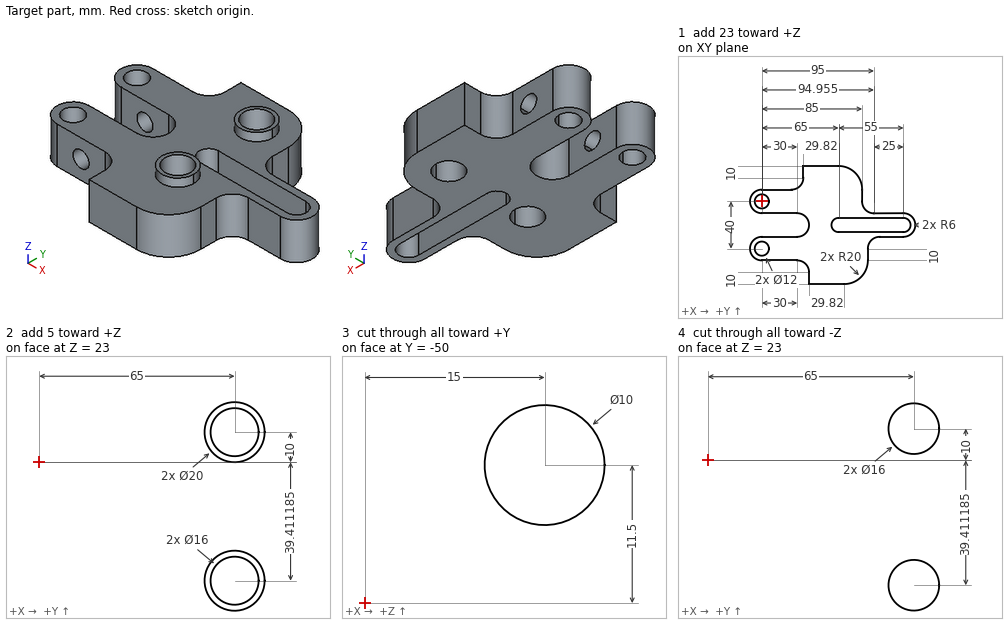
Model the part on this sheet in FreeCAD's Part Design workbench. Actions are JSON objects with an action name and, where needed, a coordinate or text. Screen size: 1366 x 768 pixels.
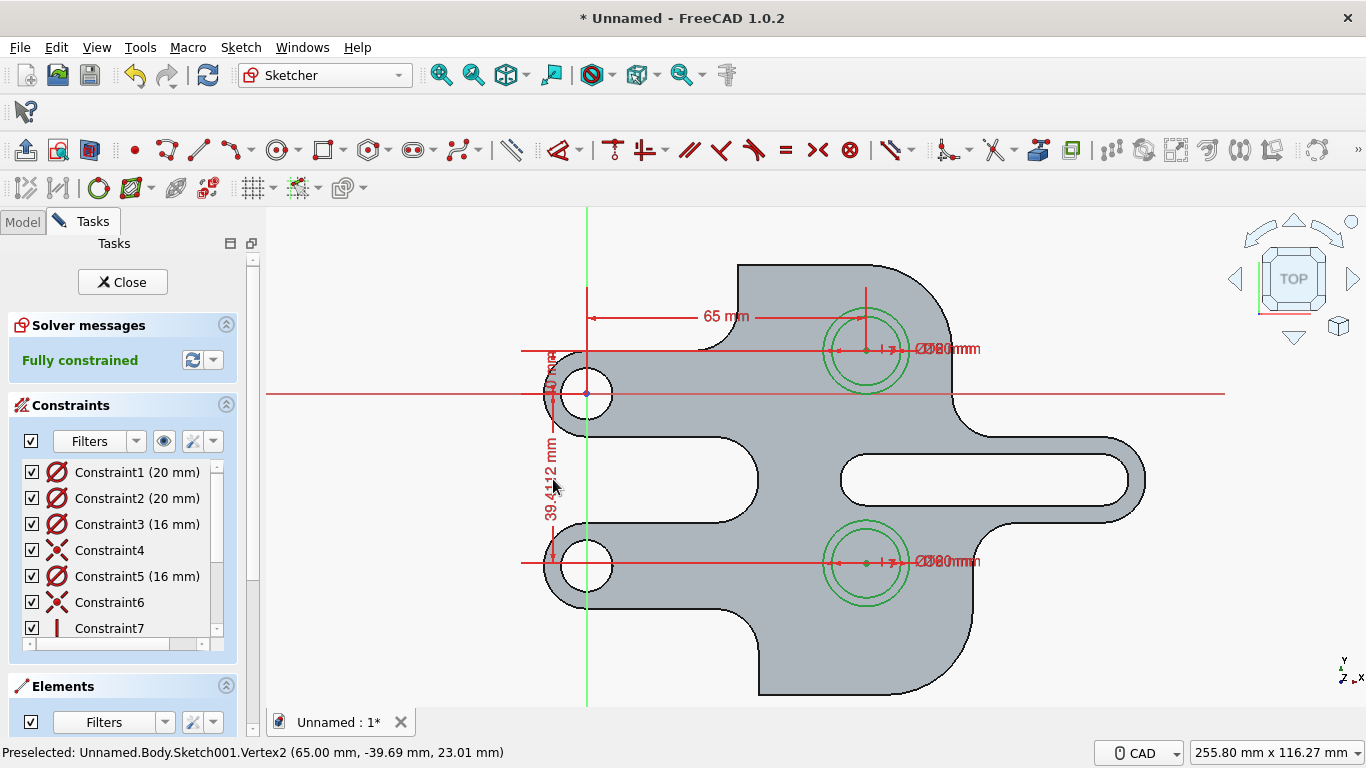
{"action": "left_click", "coordinate": [123, 282]}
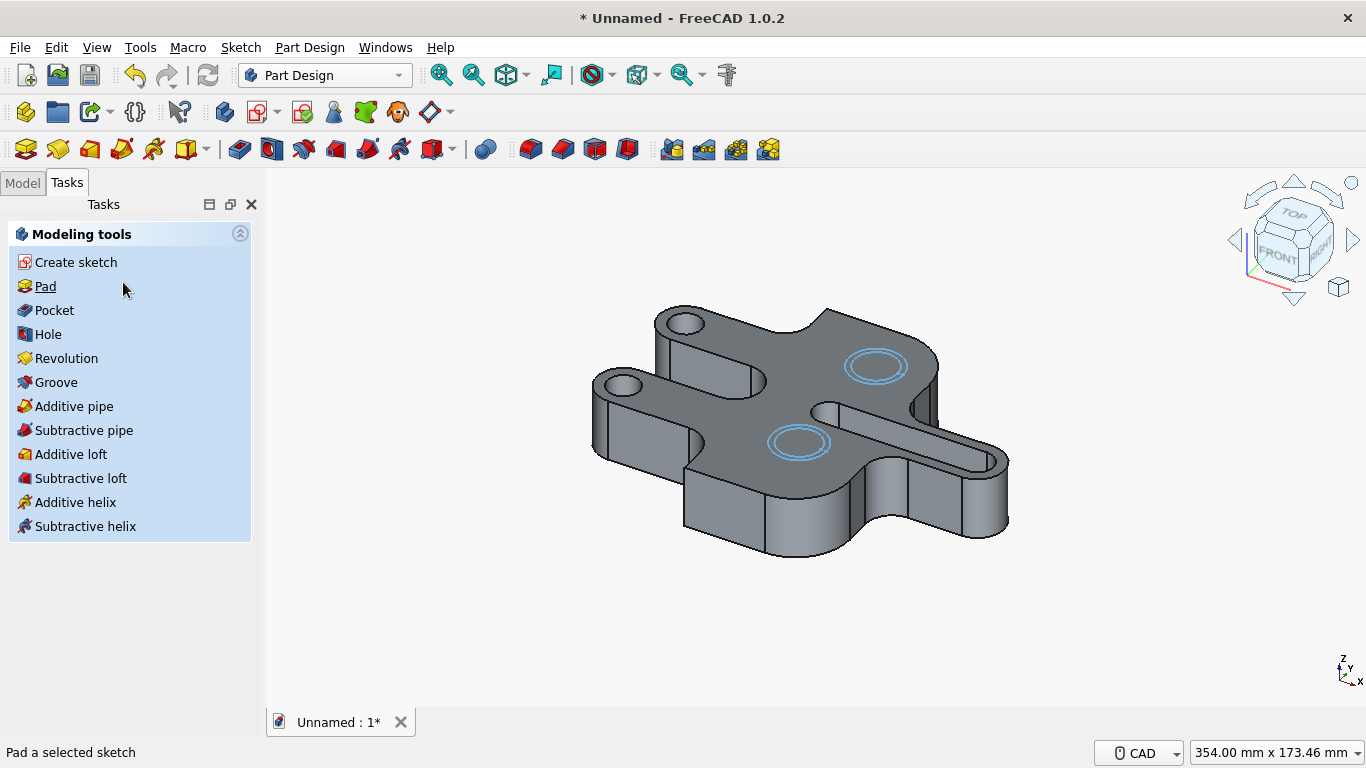
{"action": "left_click", "coordinate": [26, 150]}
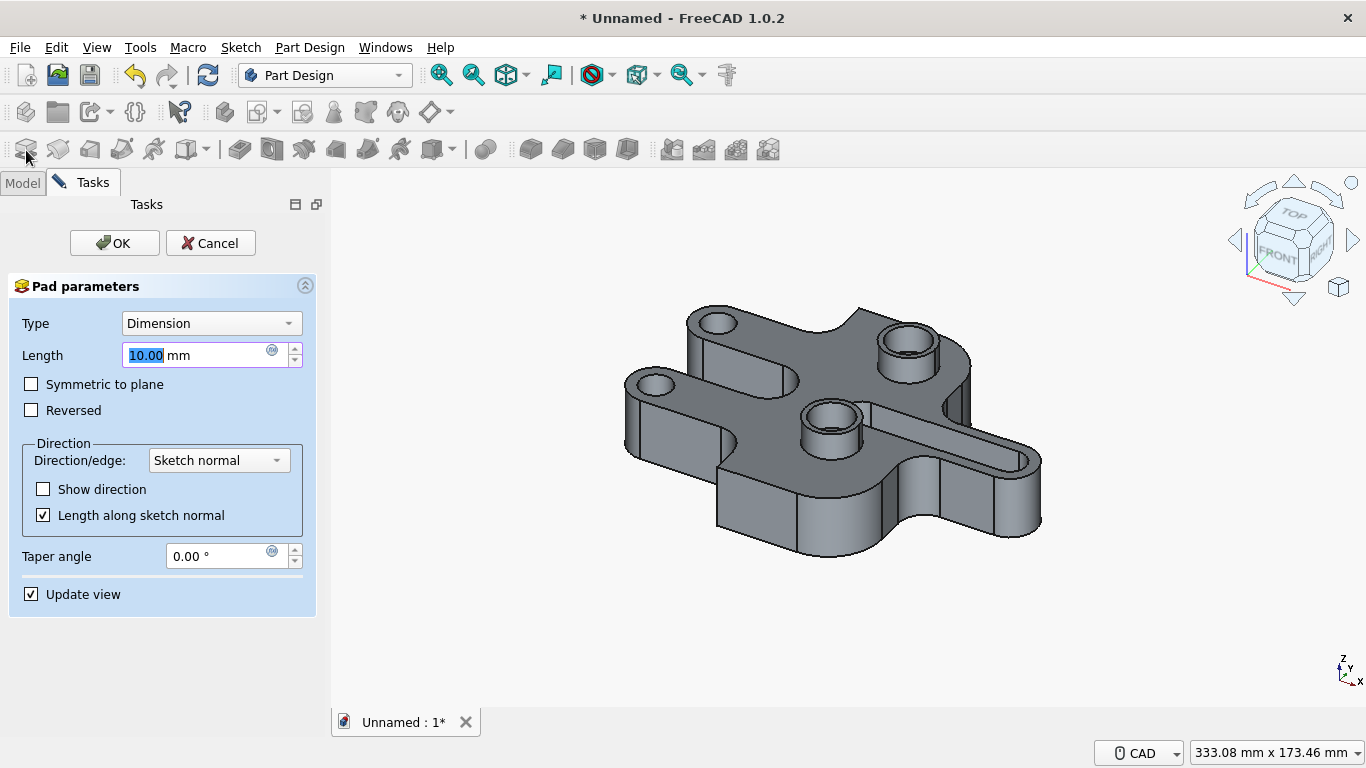
{"action": "type", "text": "5"}
{"action": "key", "text": "Tab"}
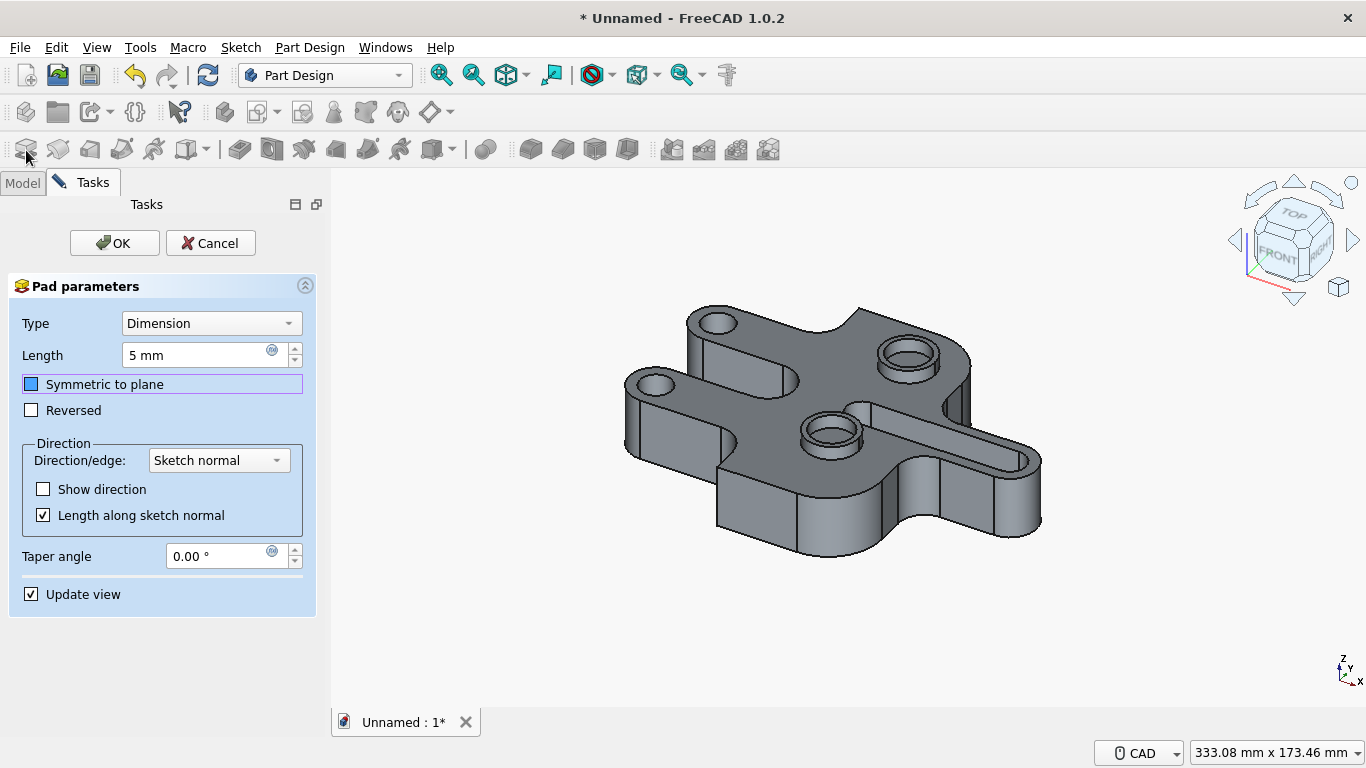
{"action": "left_click", "coordinate": [115, 243]}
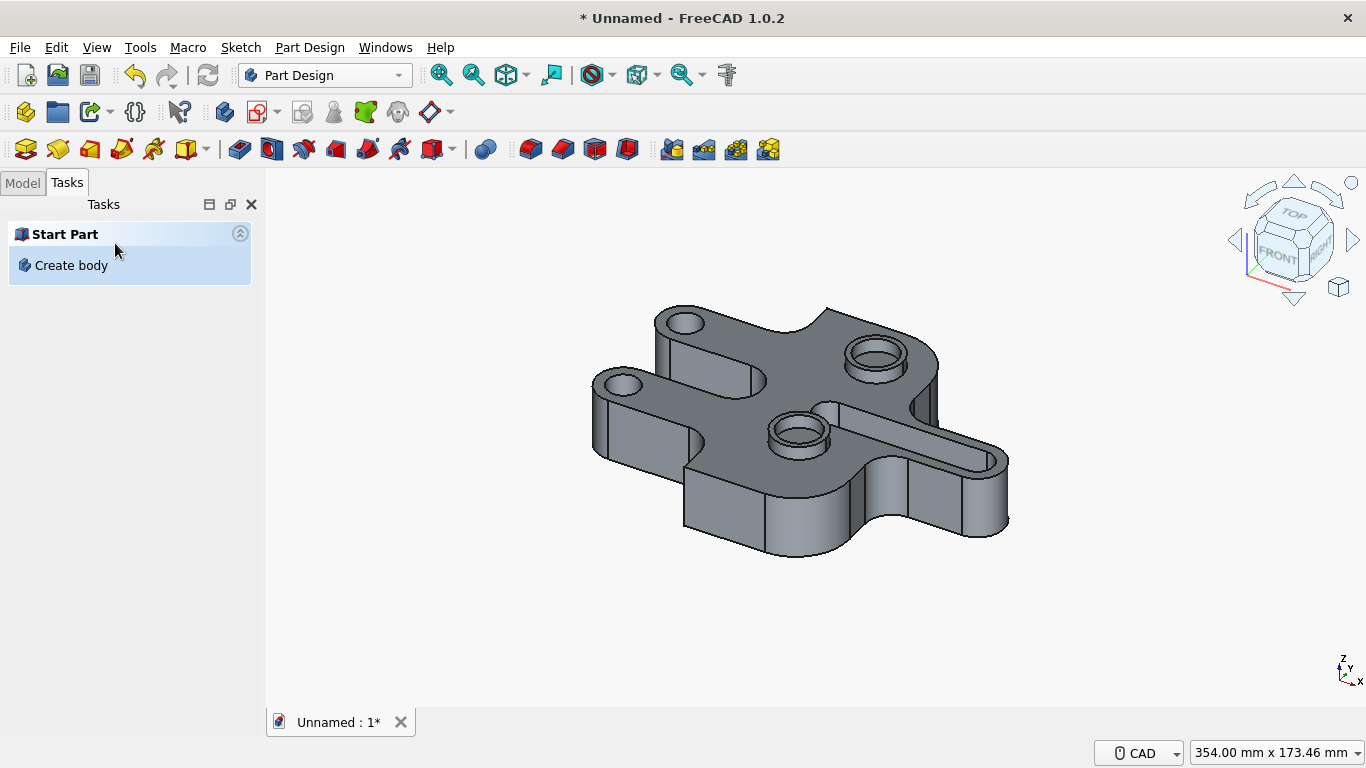
{"action": "left_click", "coordinate": [648, 442]}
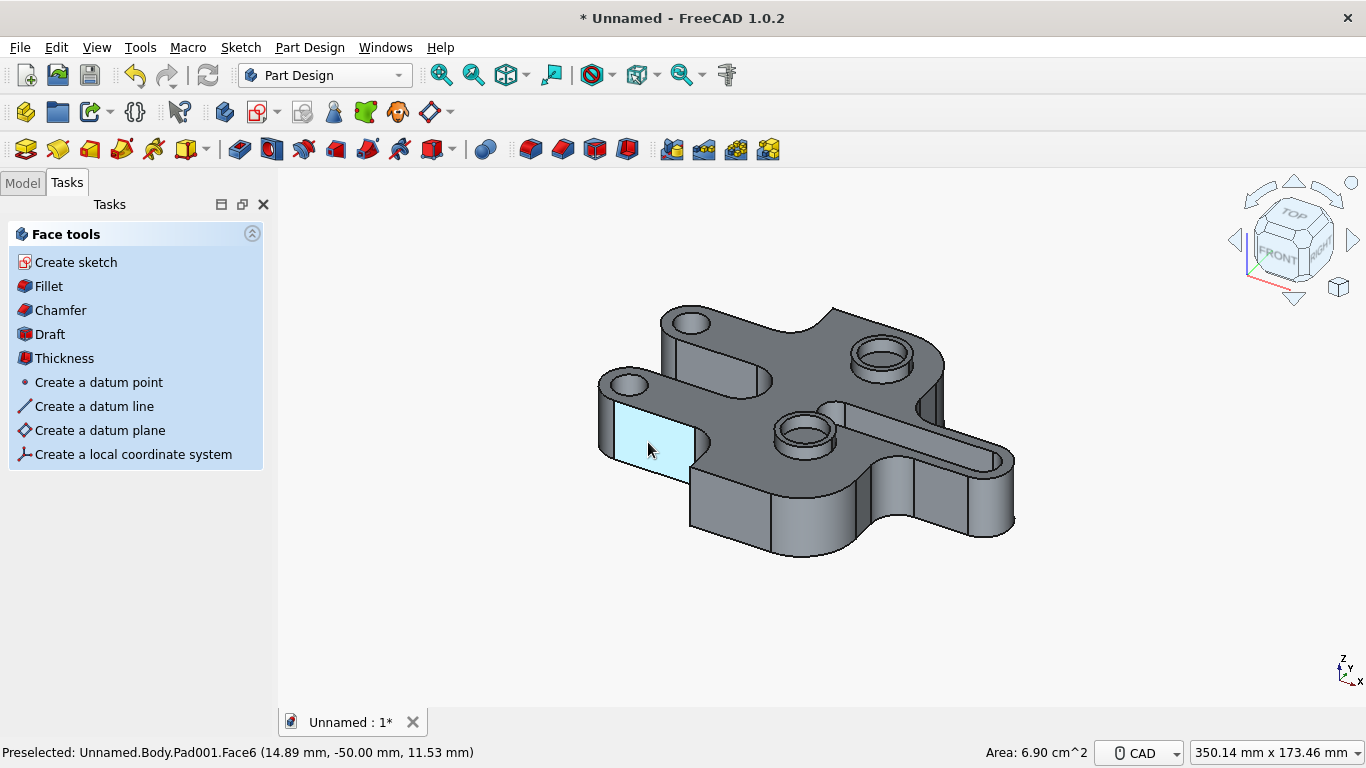
{"action": "left_click", "coordinate": [258, 112]}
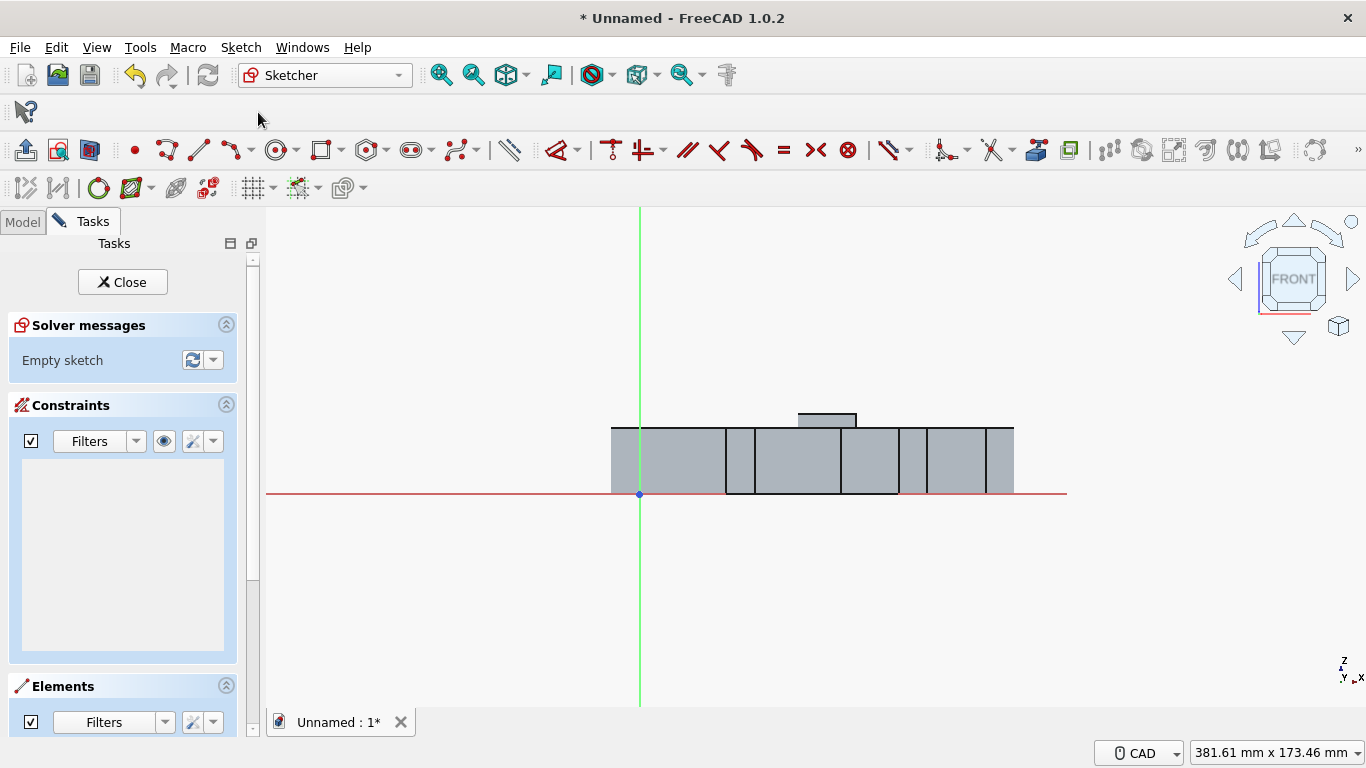
{"action": "scroll", "coordinate": [653, 473], "scroll_direction": "up", "scroll_amount": 9}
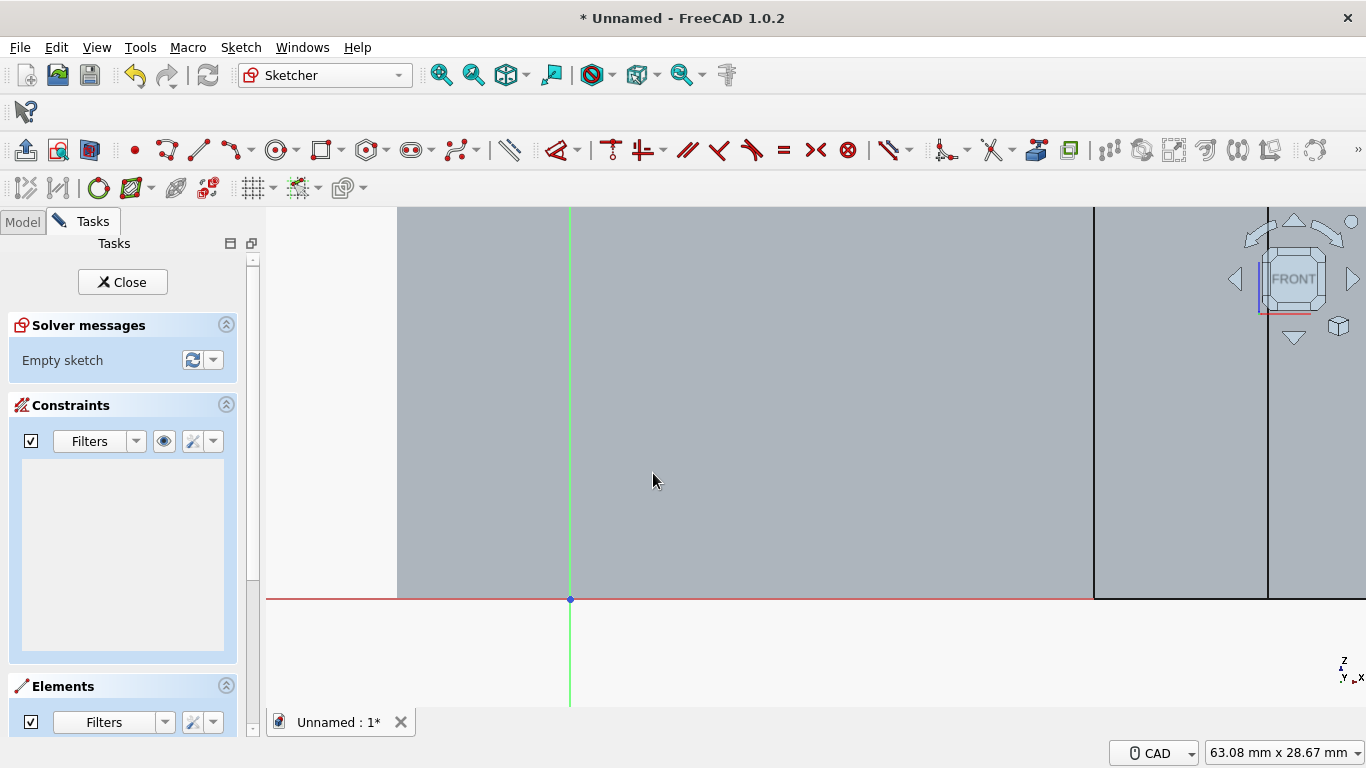
{"action": "left_click", "coordinate": [276, 150]}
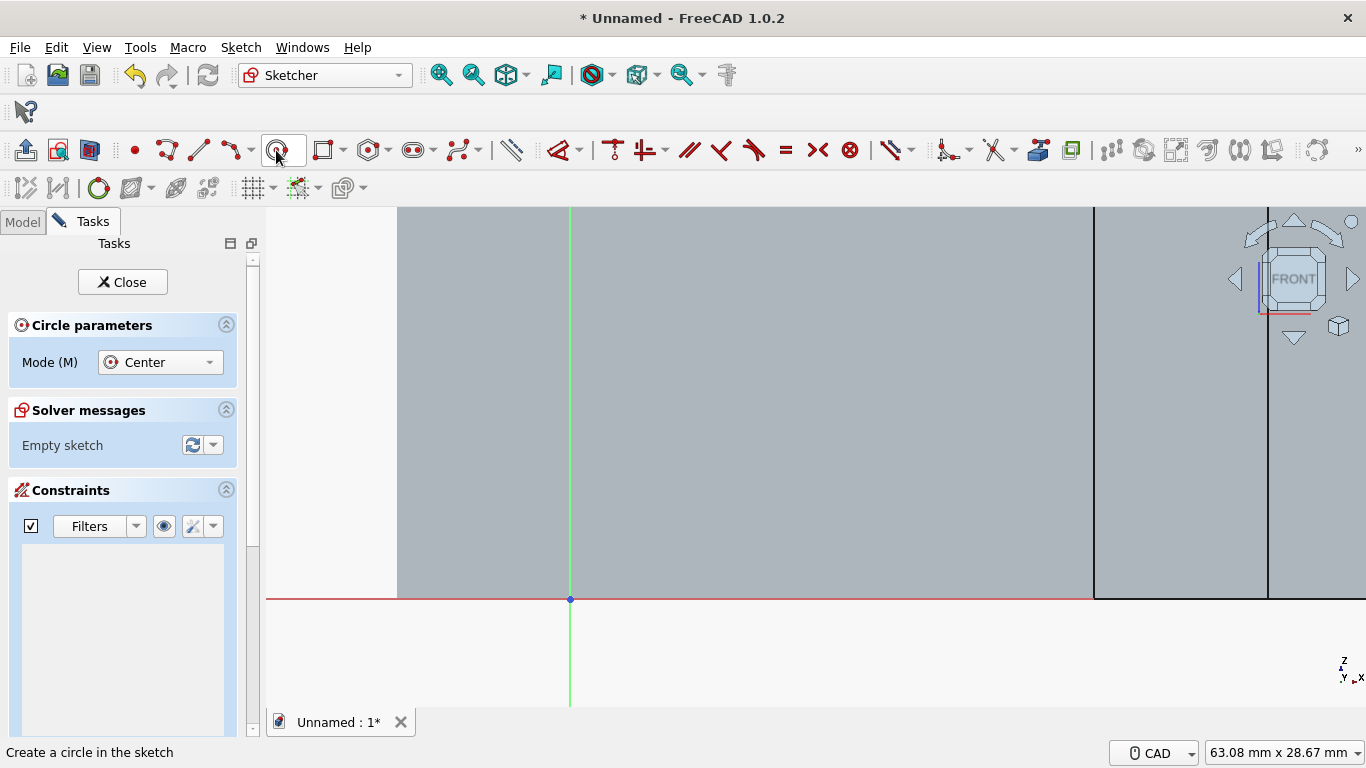
{"action": "left_click", "coordinate": [832, 399]}
{"action": "mouse_move", "coordinate": [894, 337]}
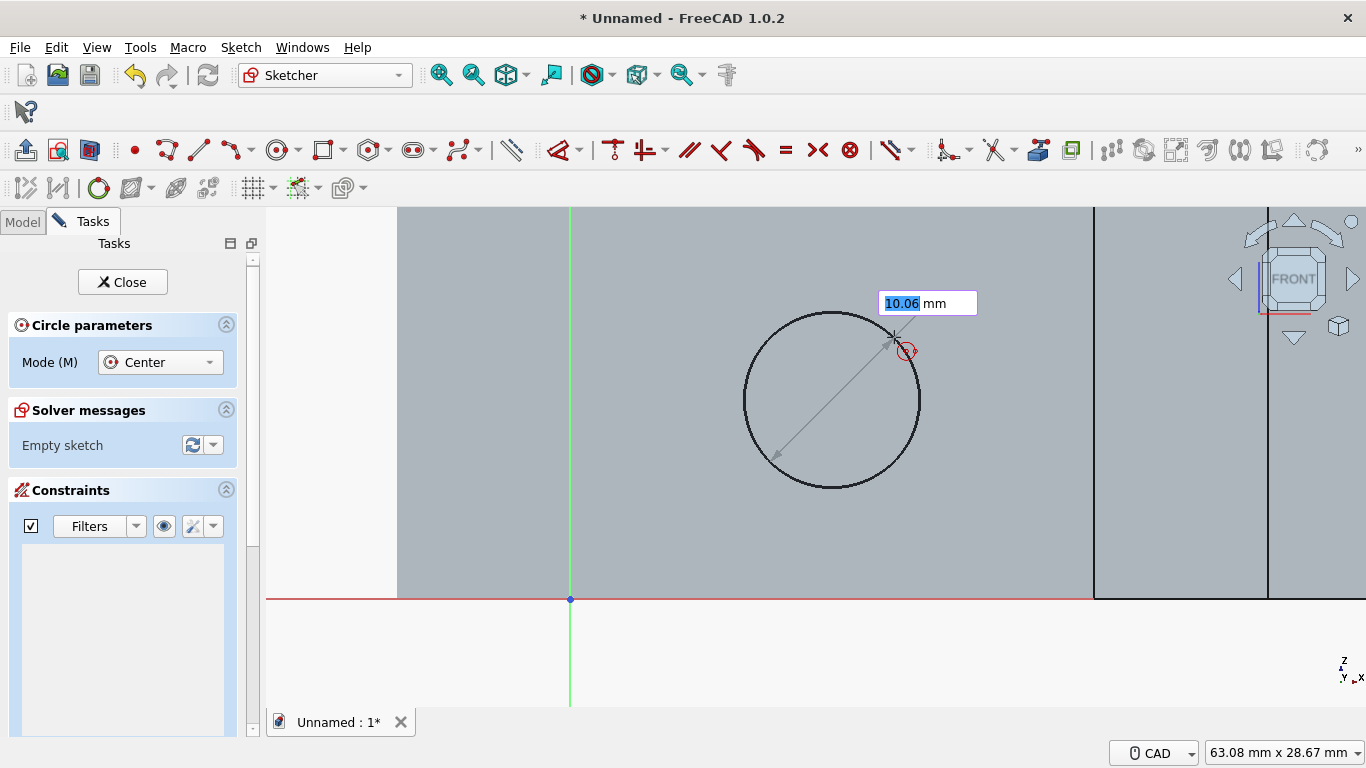
{"action": "type", "text": "10"}
{"action": "key", "text": "Return"}
{"action": "key", "text": "Escape"}